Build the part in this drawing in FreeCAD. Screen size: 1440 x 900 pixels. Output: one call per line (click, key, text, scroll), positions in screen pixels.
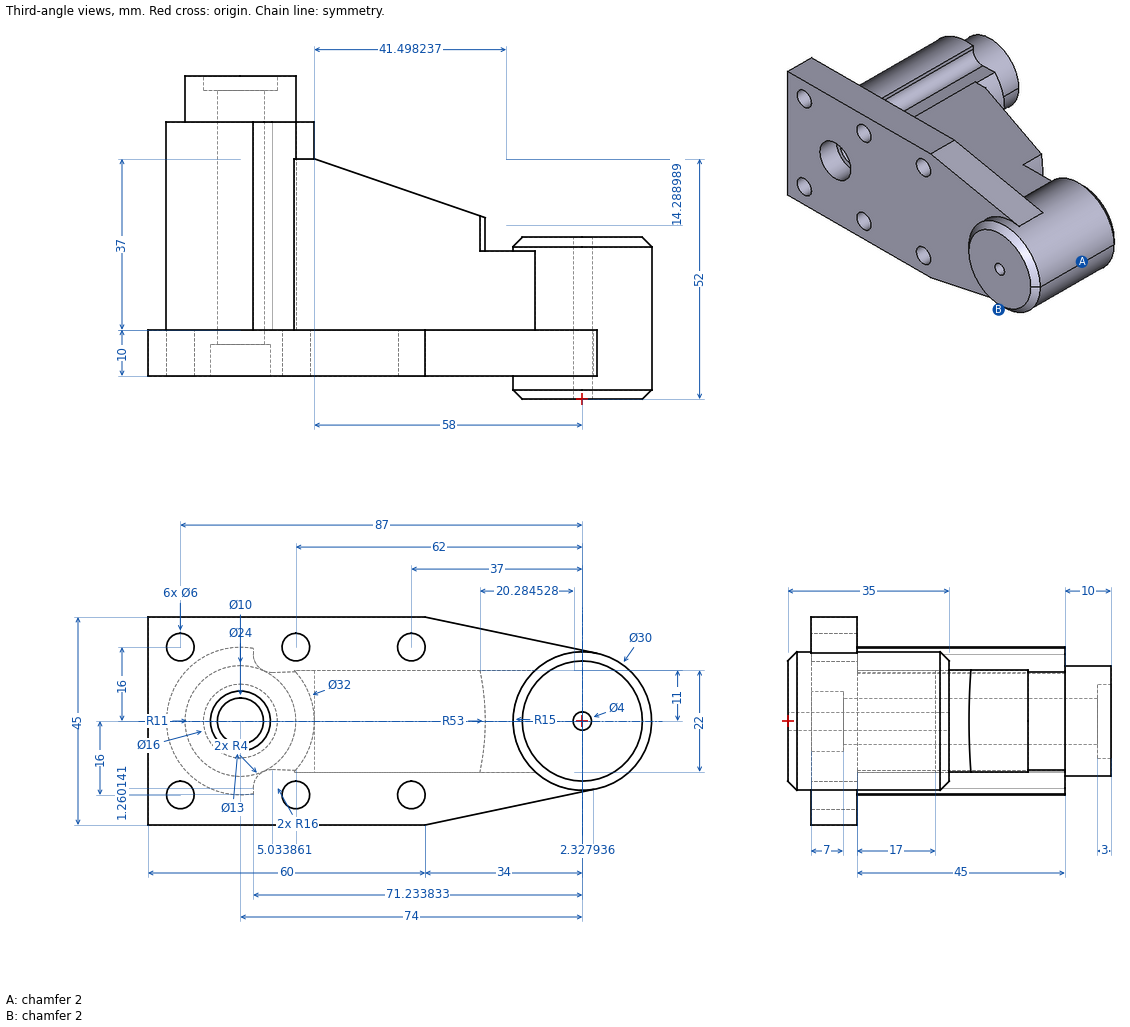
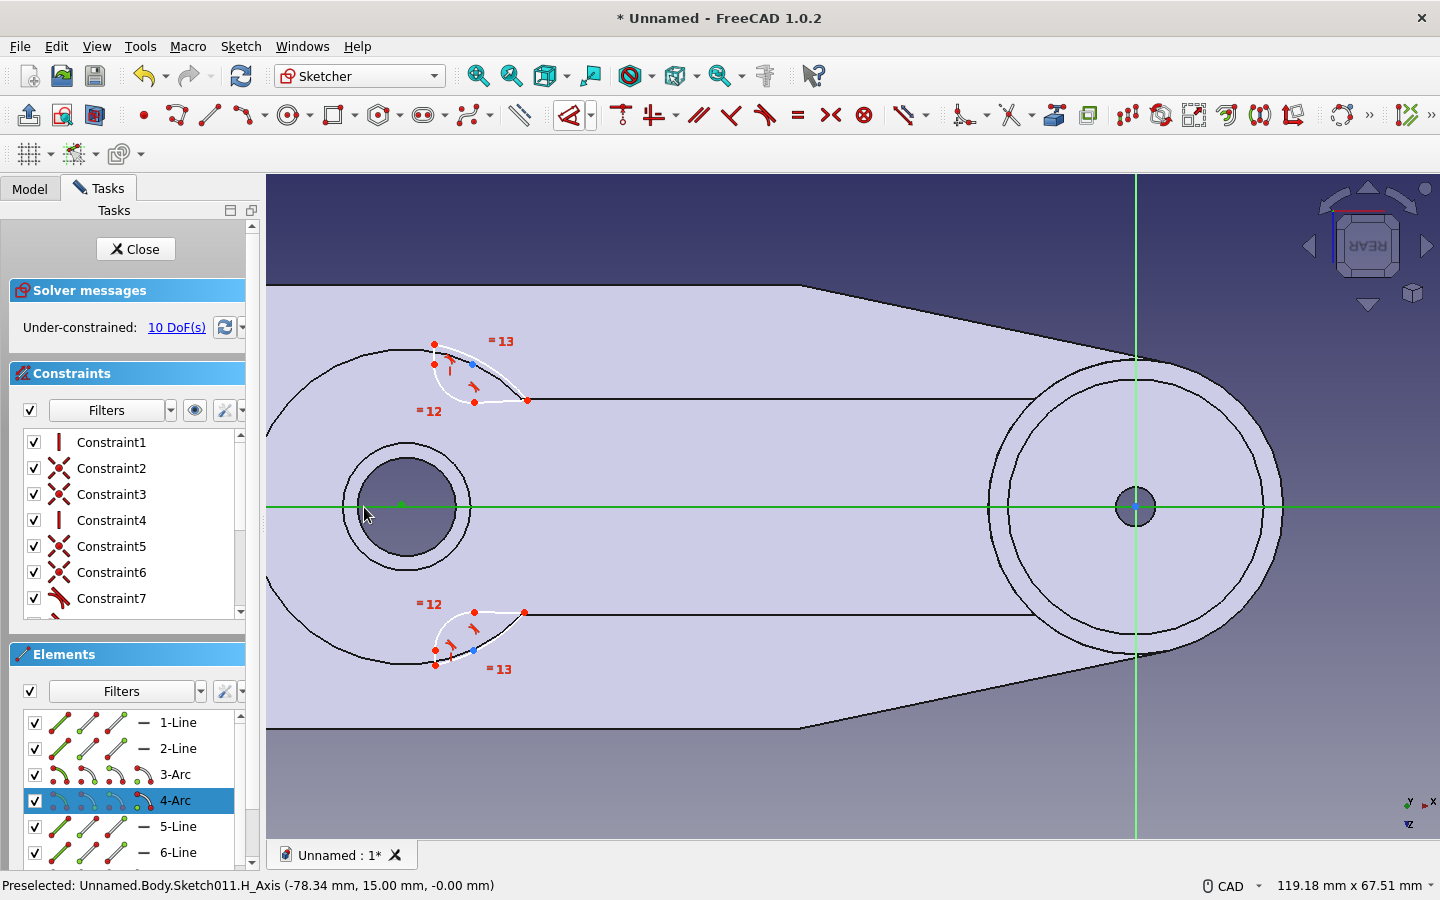
click(621, 116)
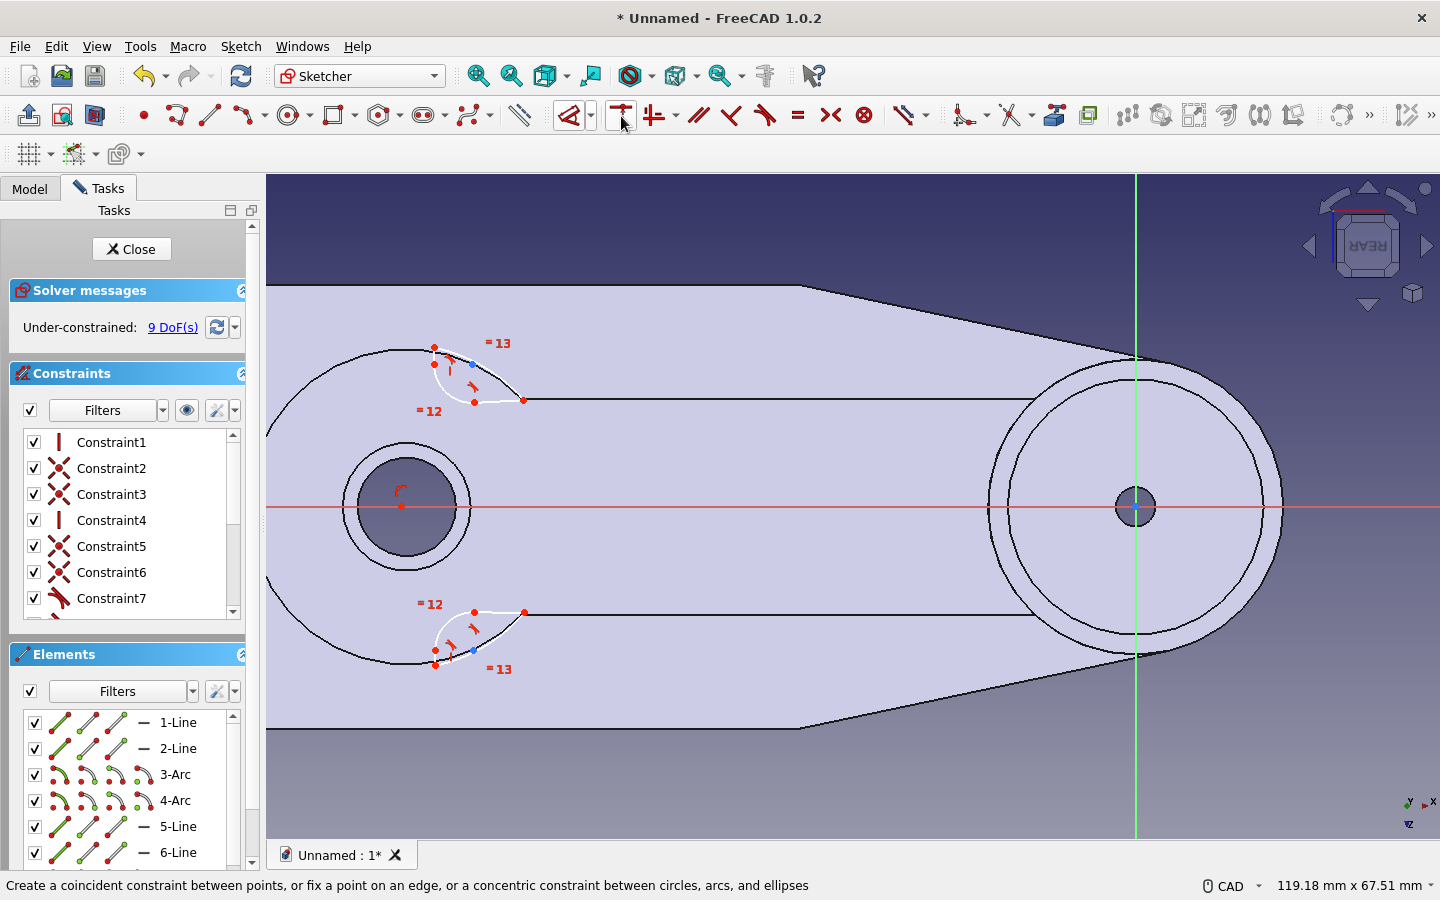
click(473, 364)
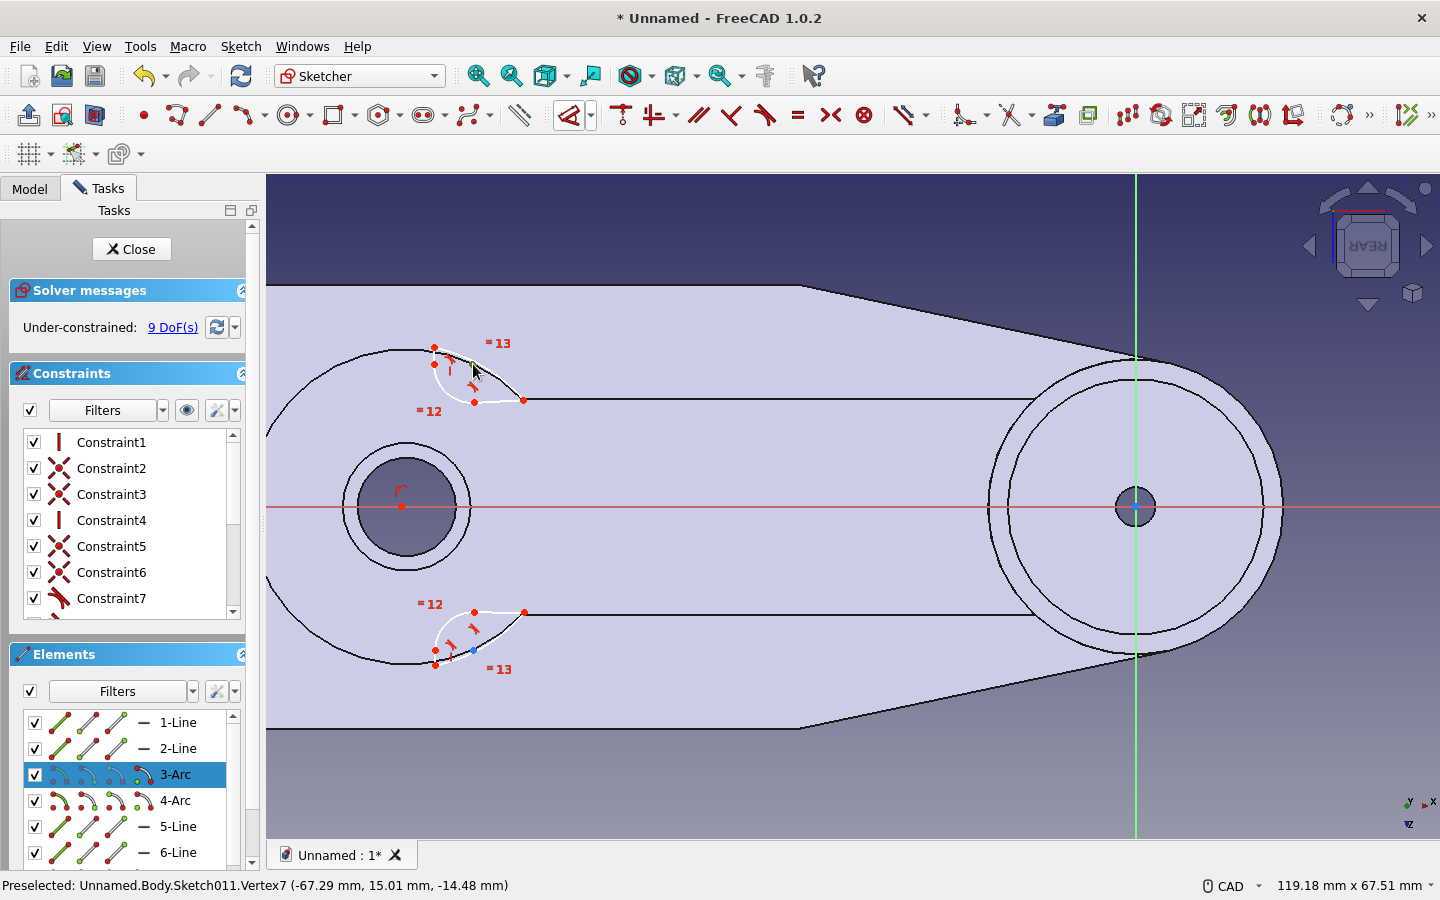
click(474, 651)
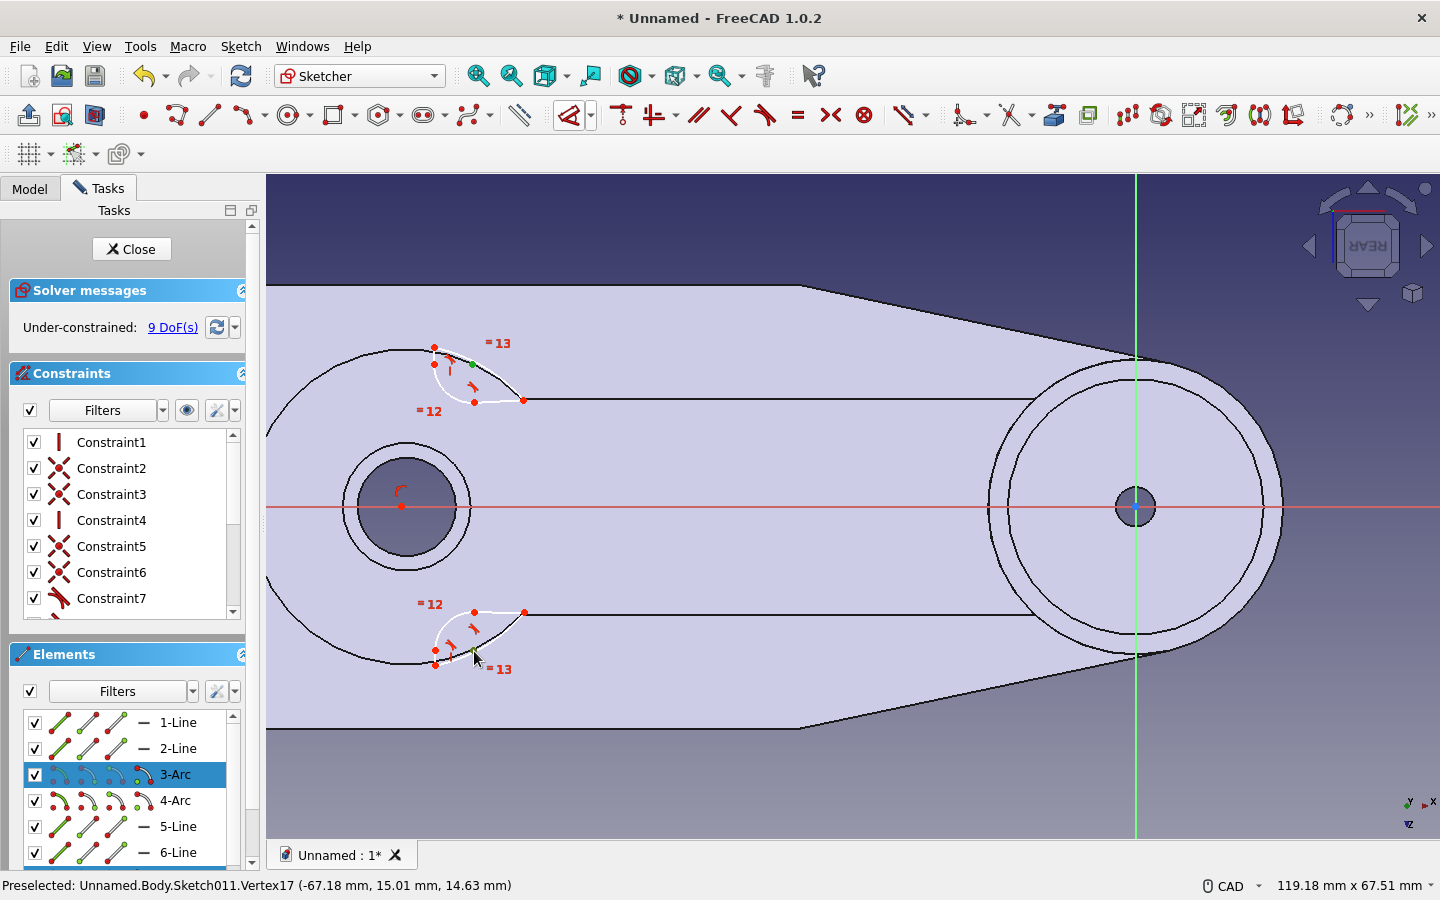
click(364, 507)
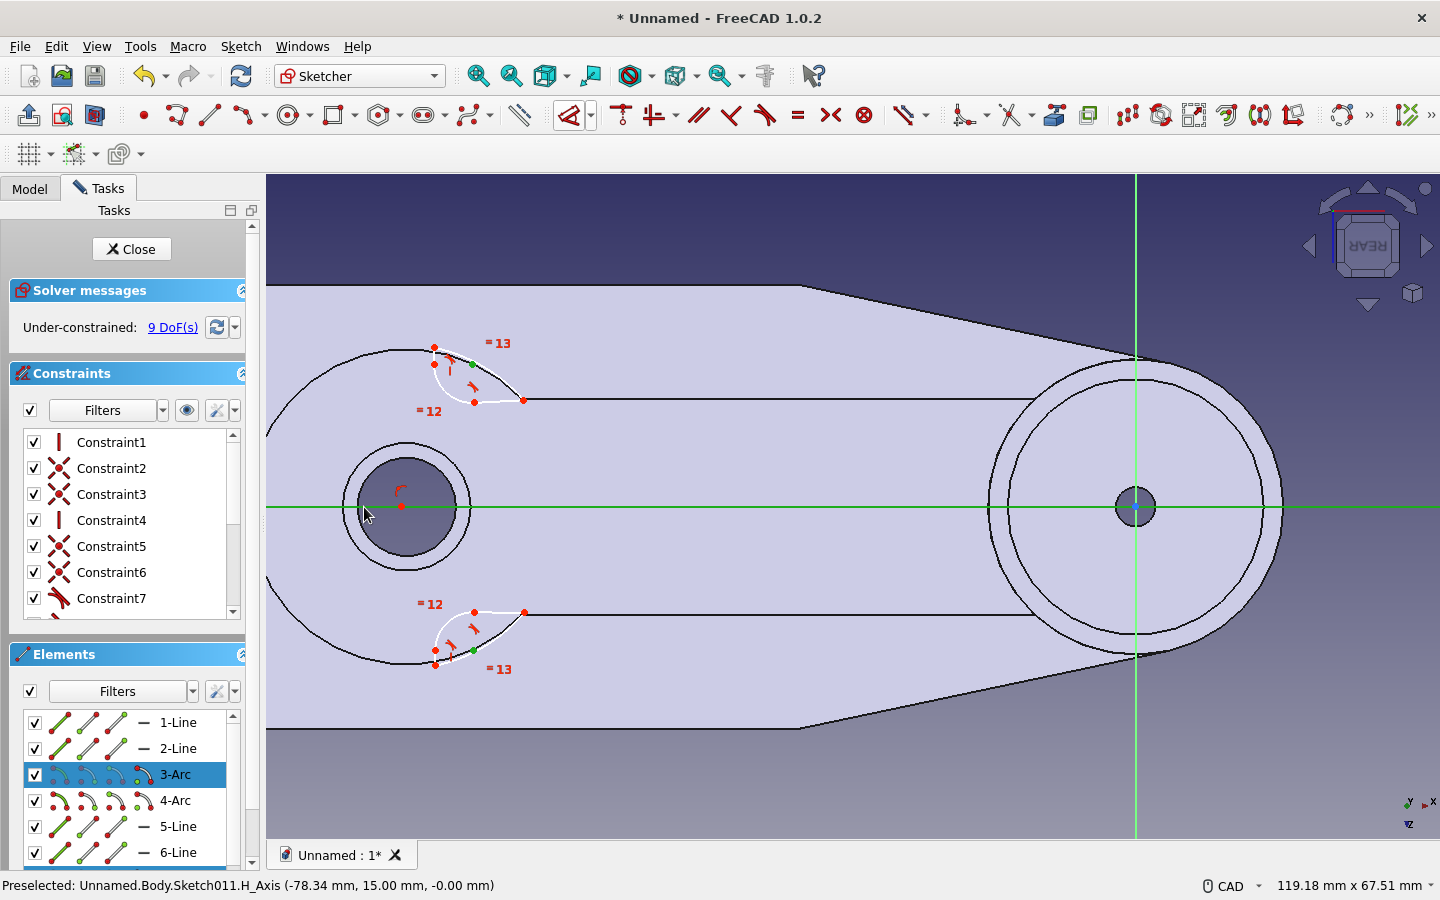
click(831, 116)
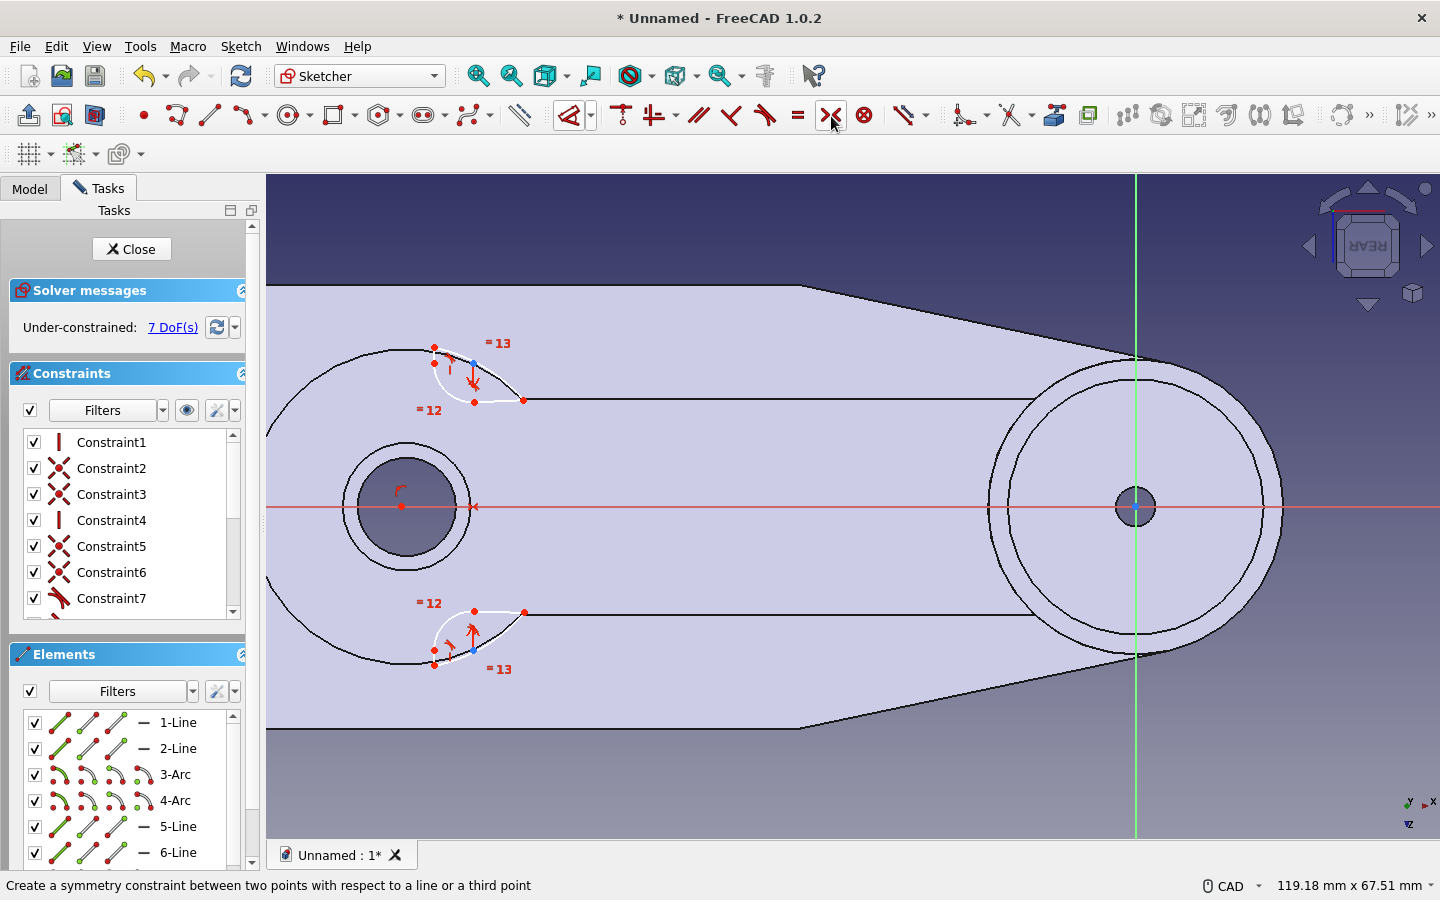
click(439, 381)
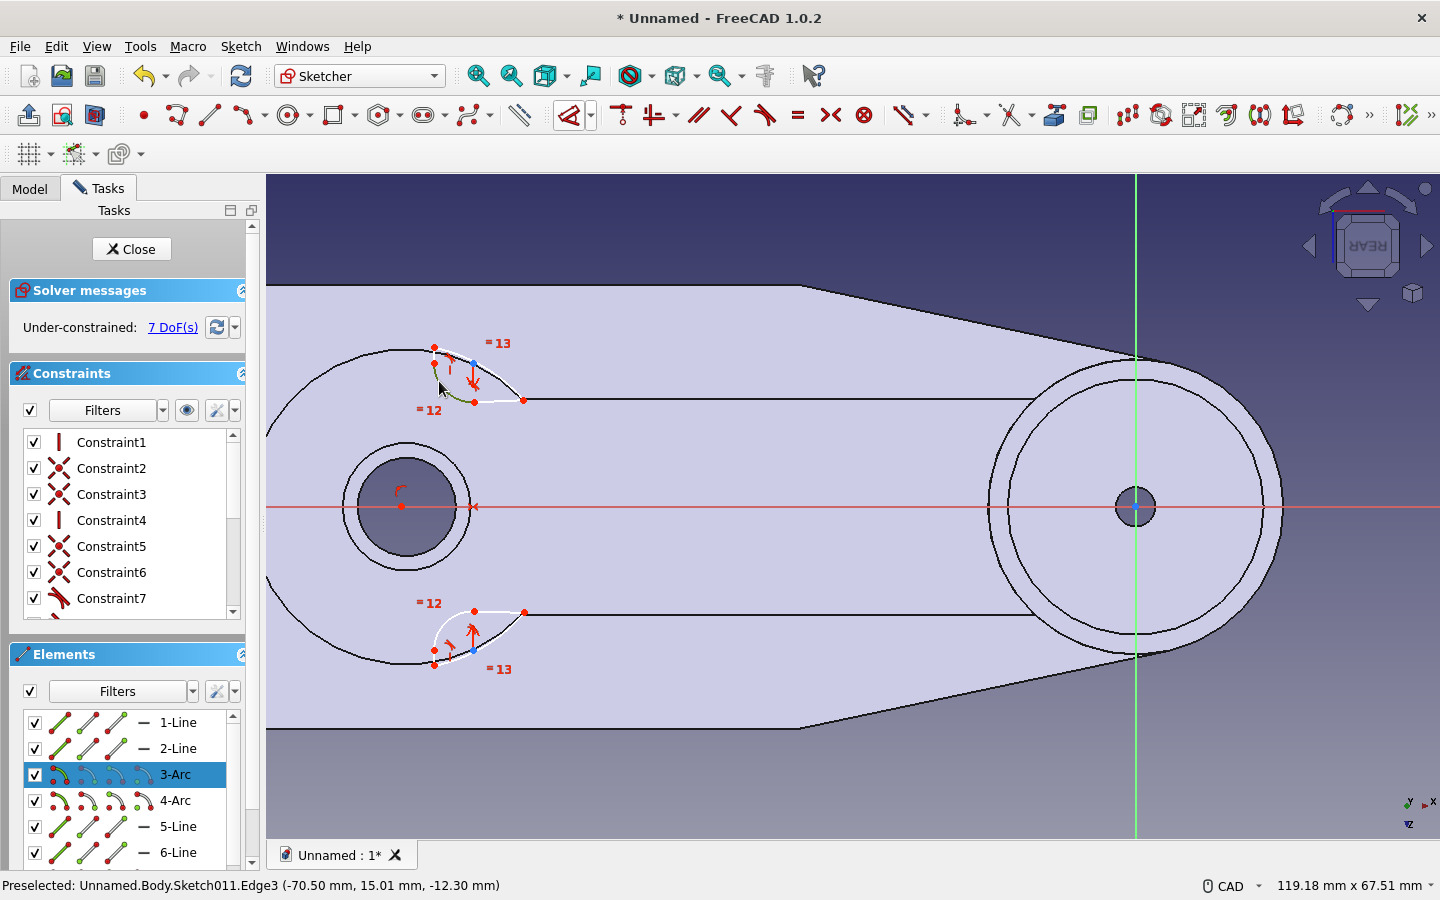
key(k)
key(r)